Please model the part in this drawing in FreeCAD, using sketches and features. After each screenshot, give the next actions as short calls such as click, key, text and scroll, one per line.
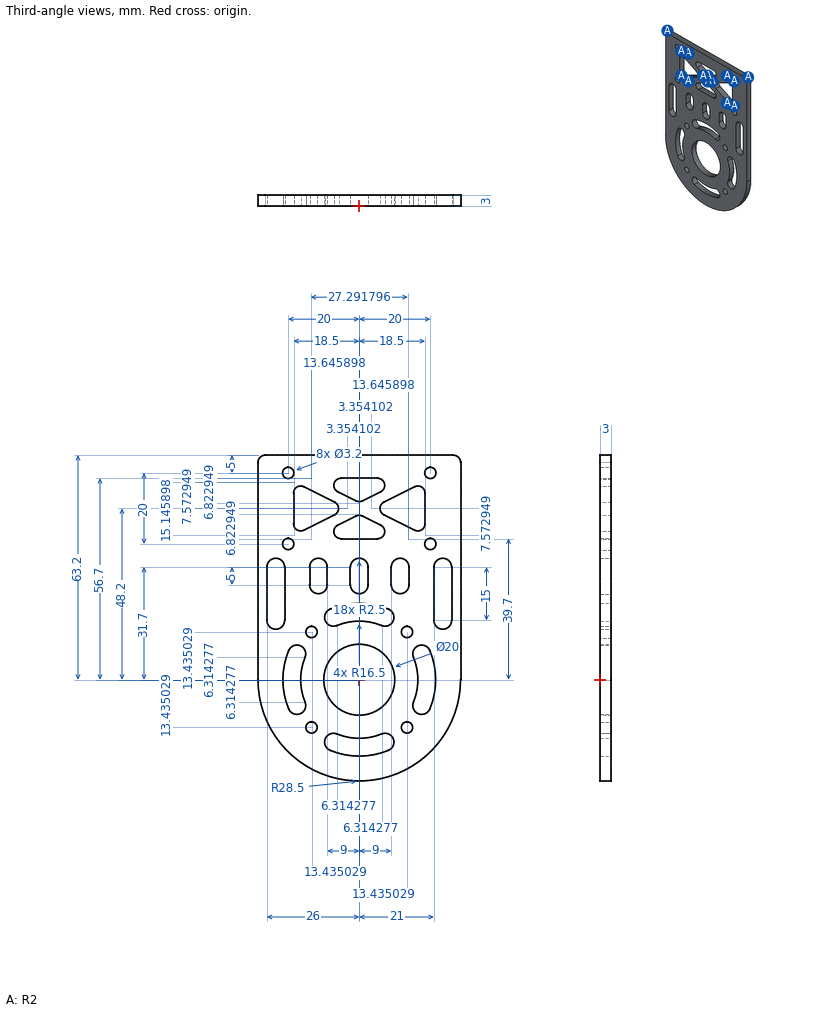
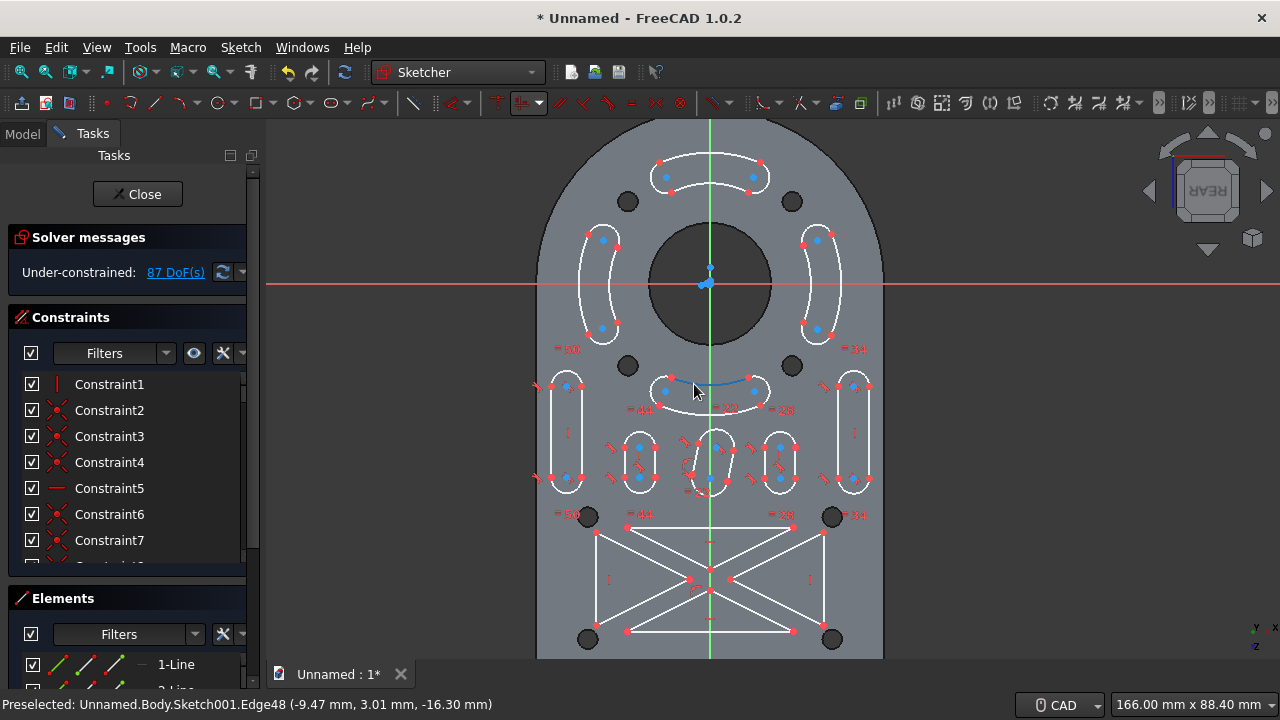
click(694, 384)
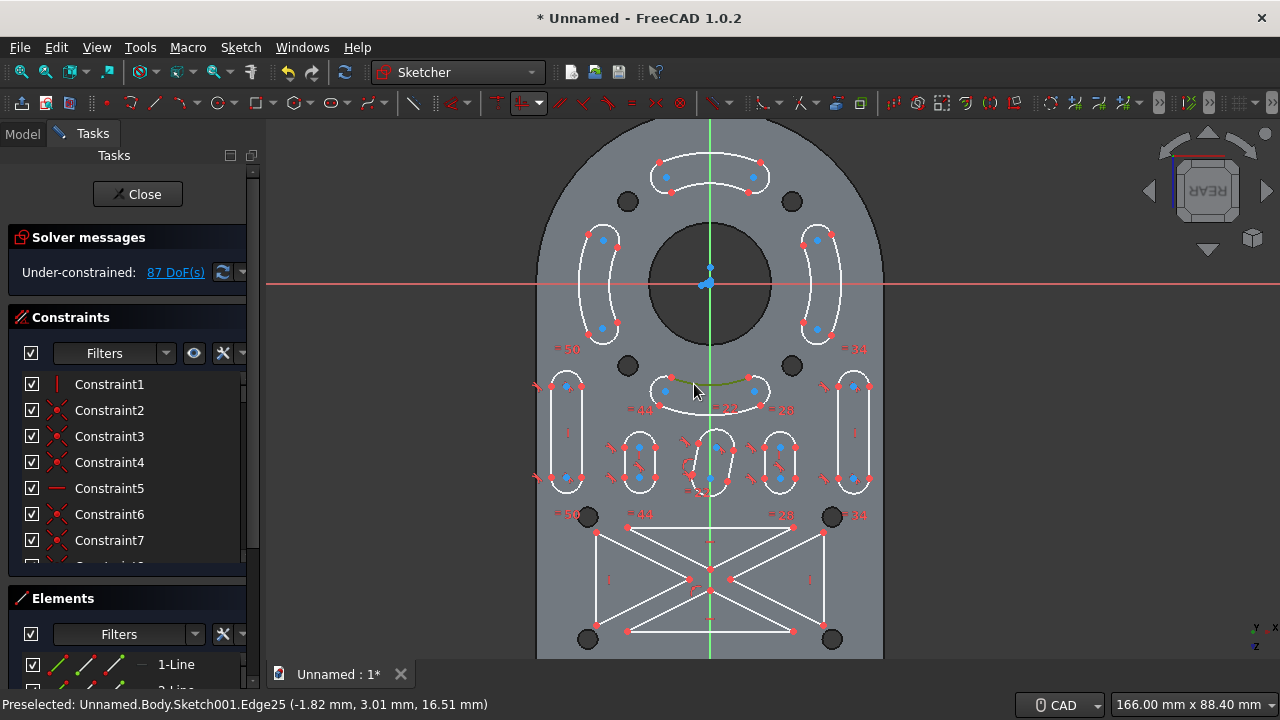
click(658, 379)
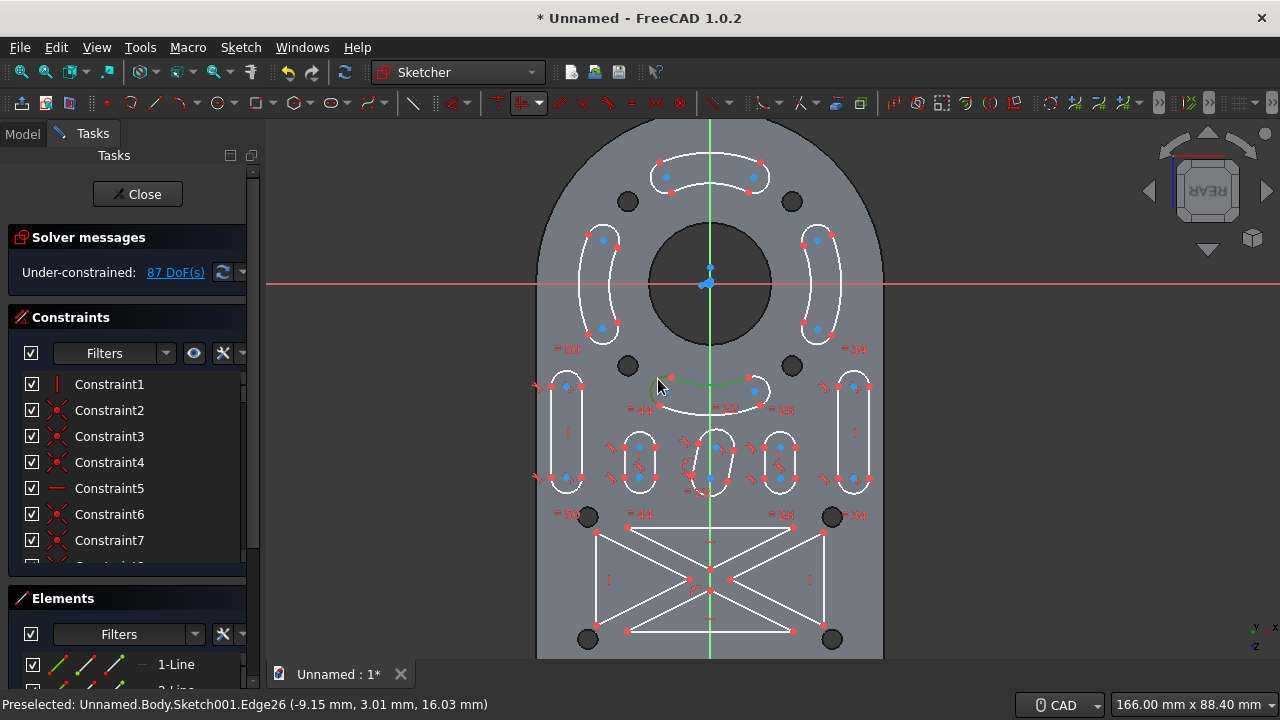
key(t)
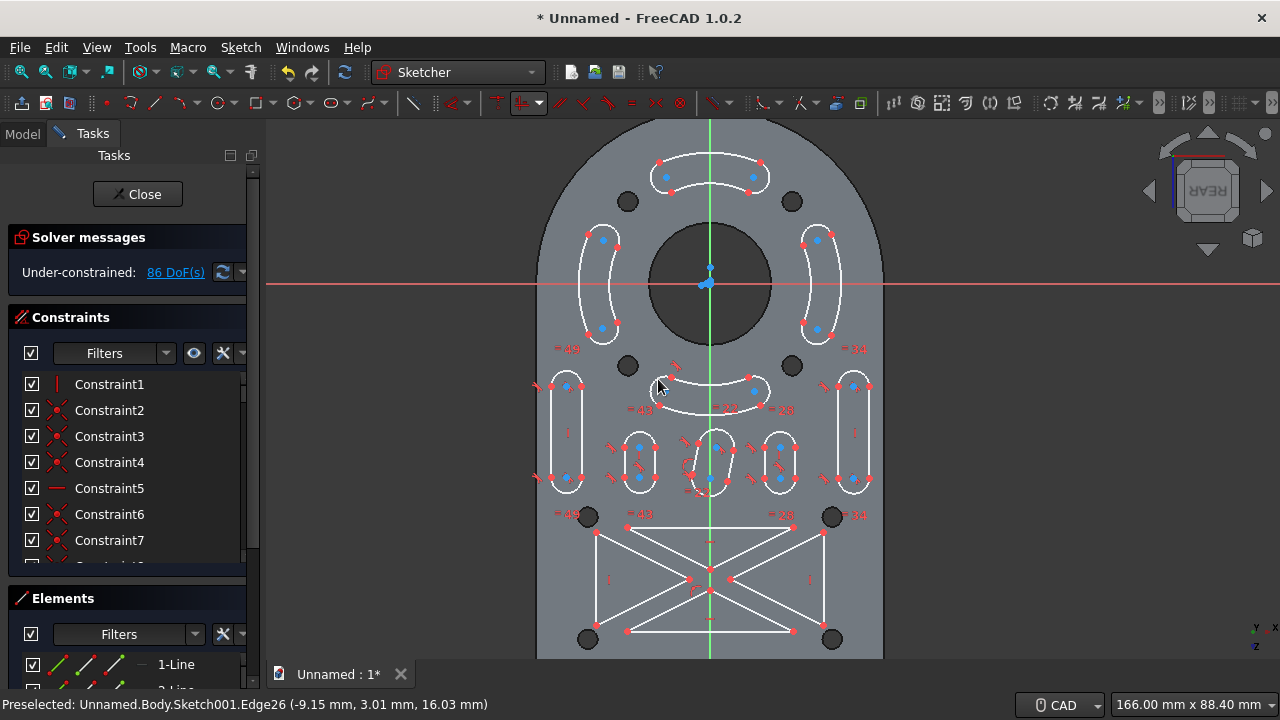
click(694, 384)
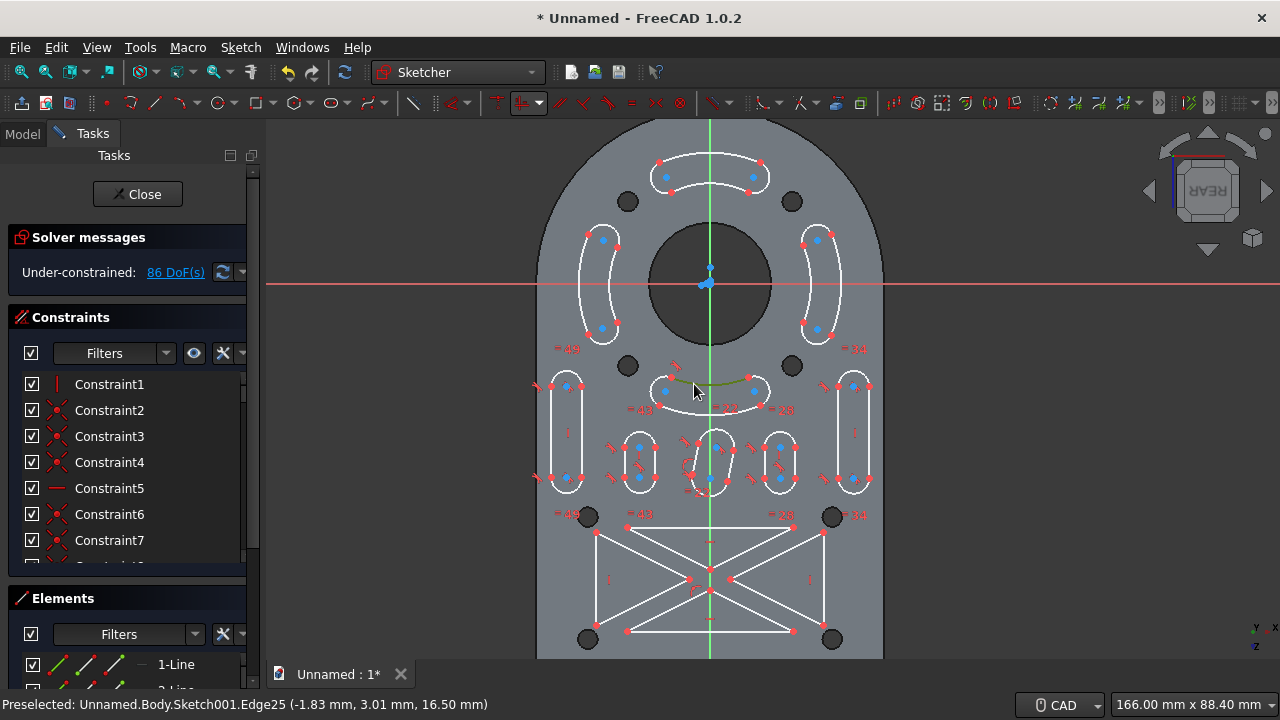
click(769, 395)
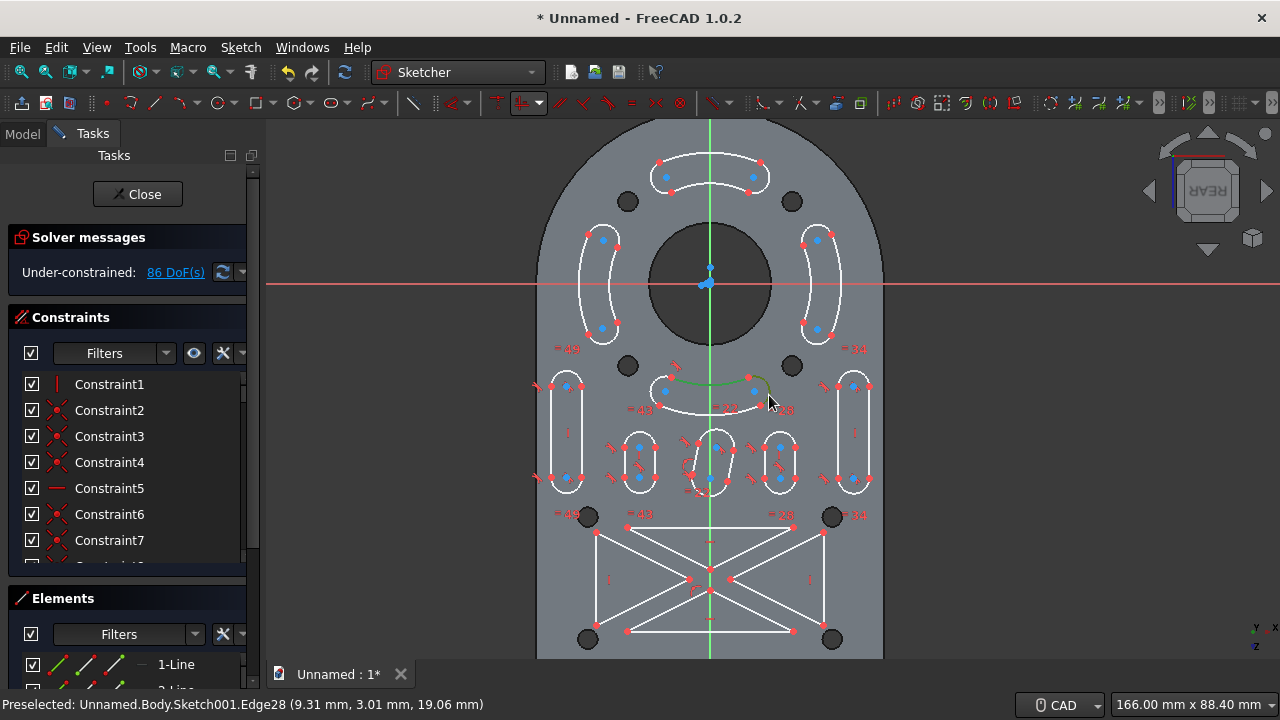
key(t)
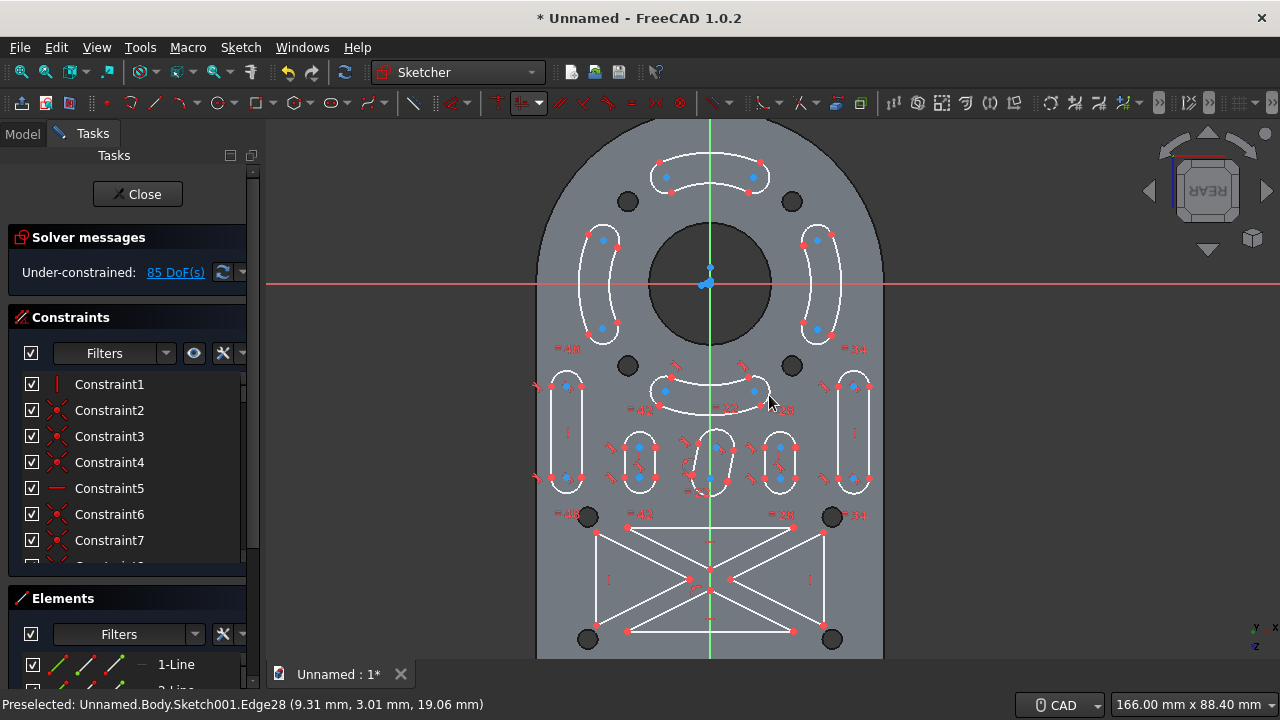
click(658, 379)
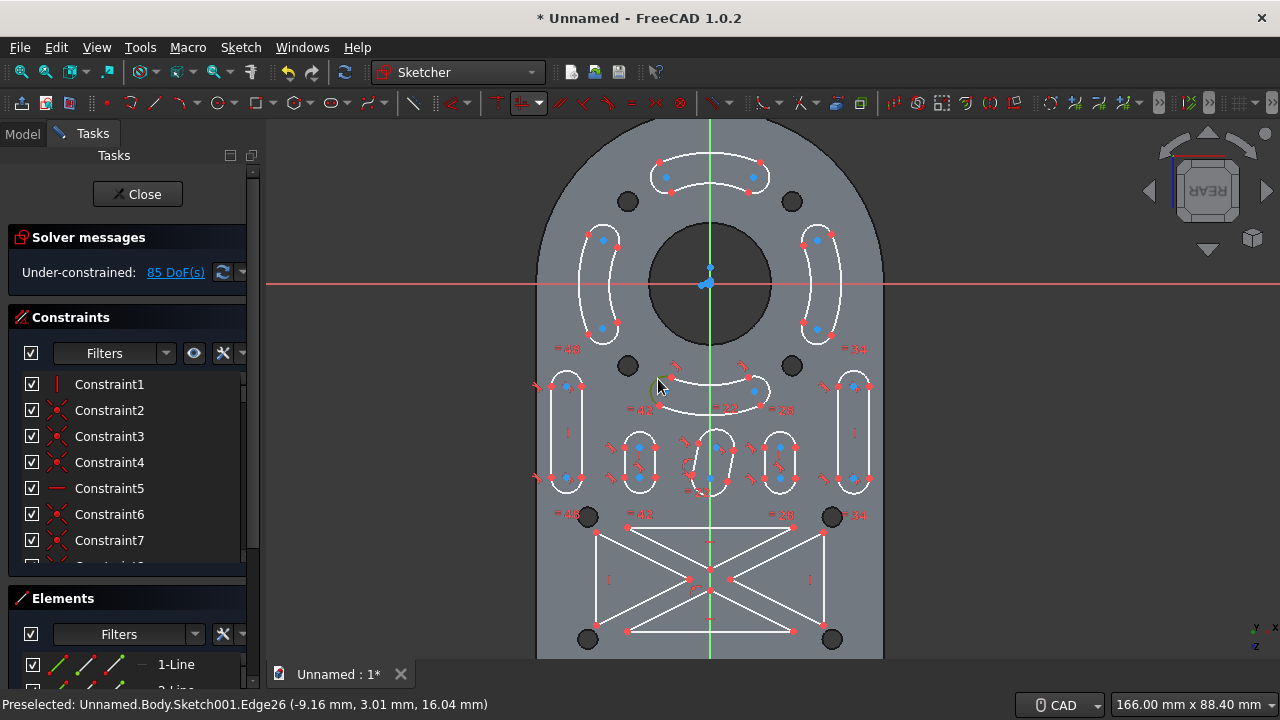
click(689, 414)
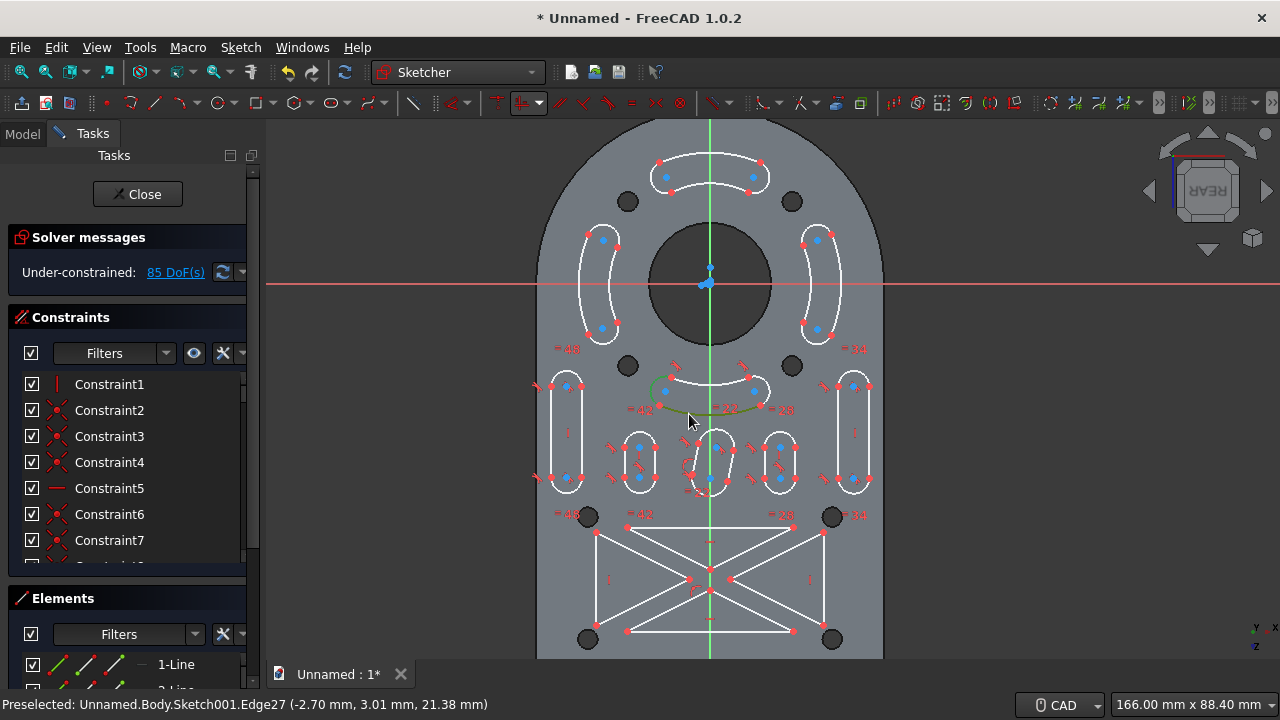
key(t)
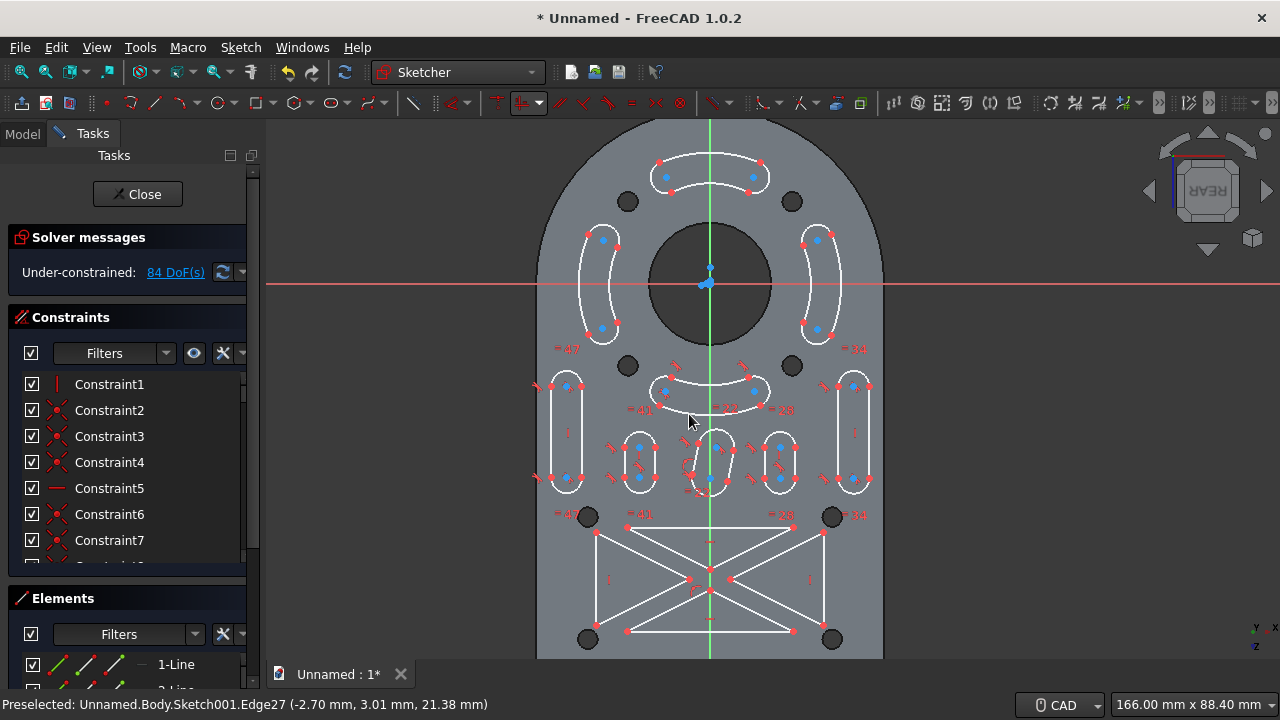
click(689, 414)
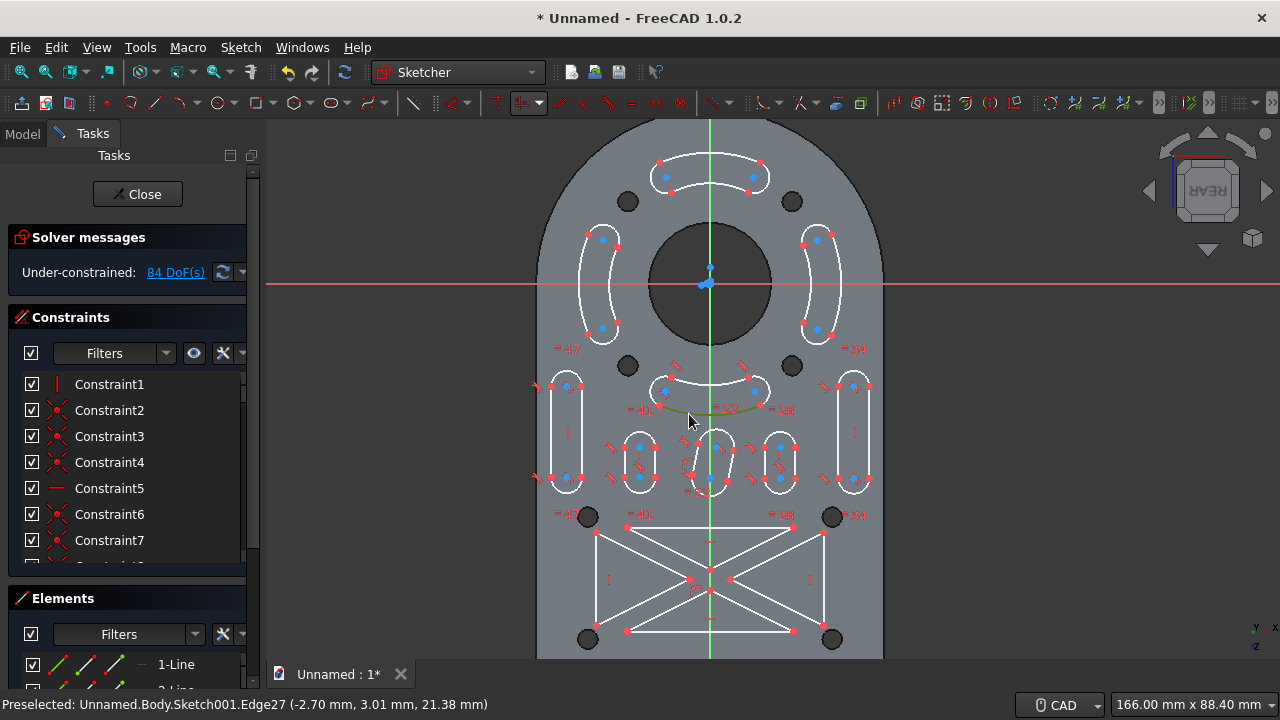
click(769, 395)